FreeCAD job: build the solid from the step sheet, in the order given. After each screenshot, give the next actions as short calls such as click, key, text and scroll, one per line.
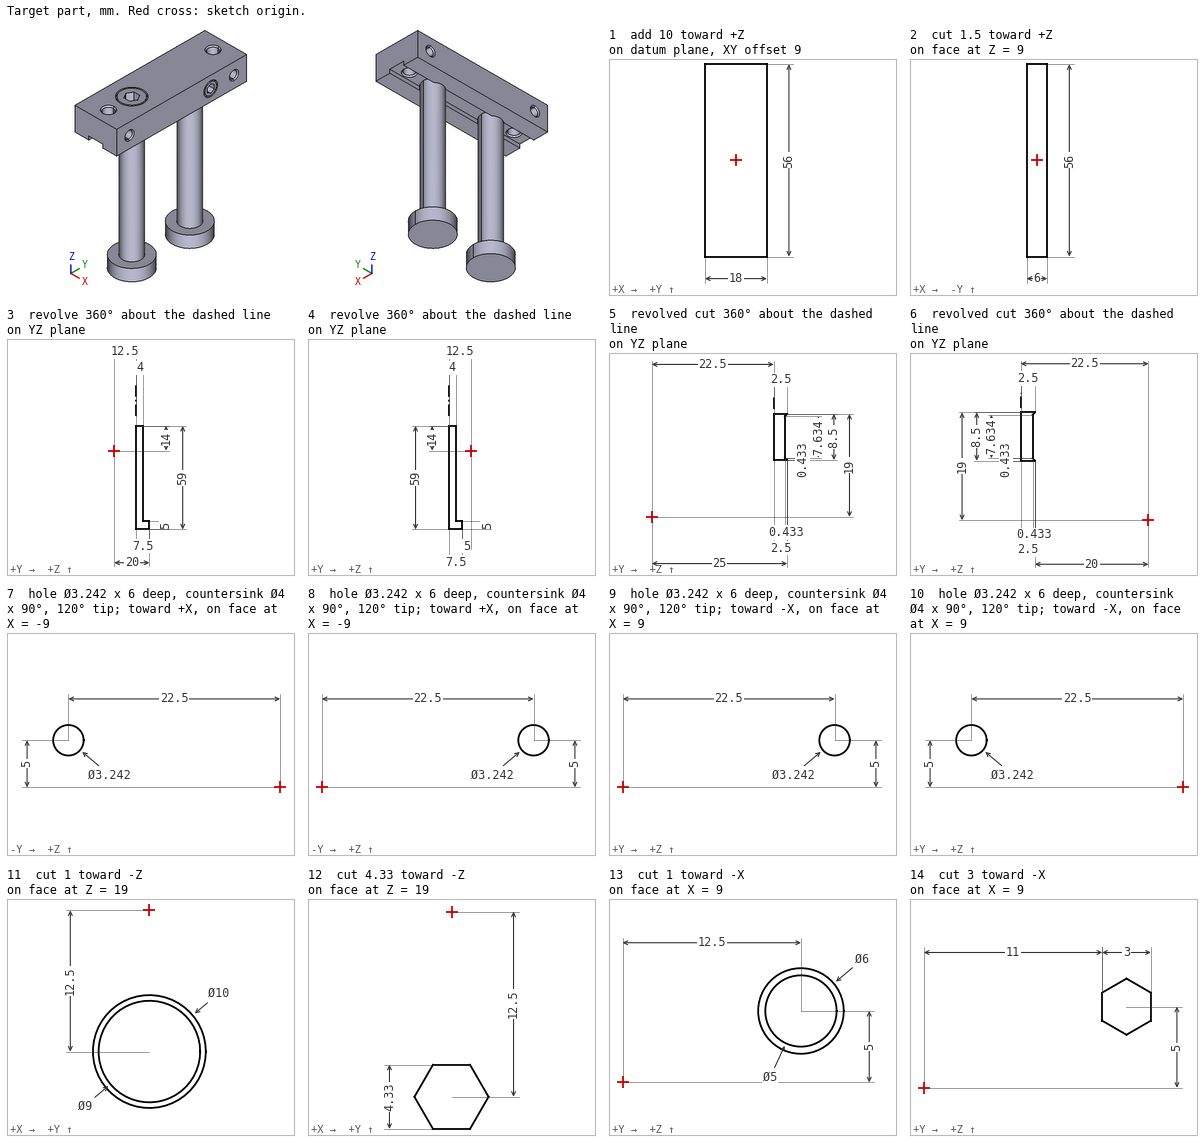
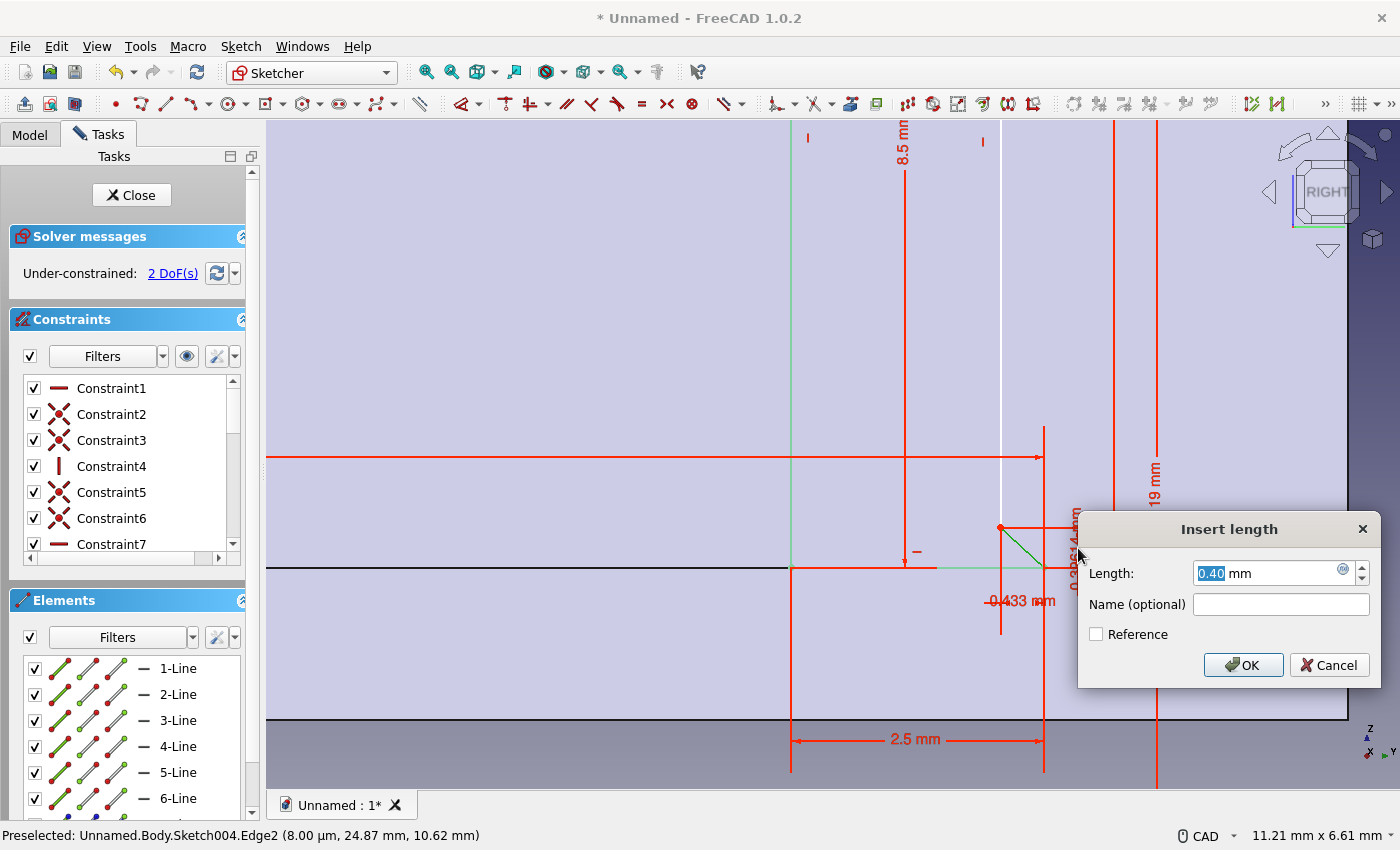
text(0.433)
key(Return)
key(Escape)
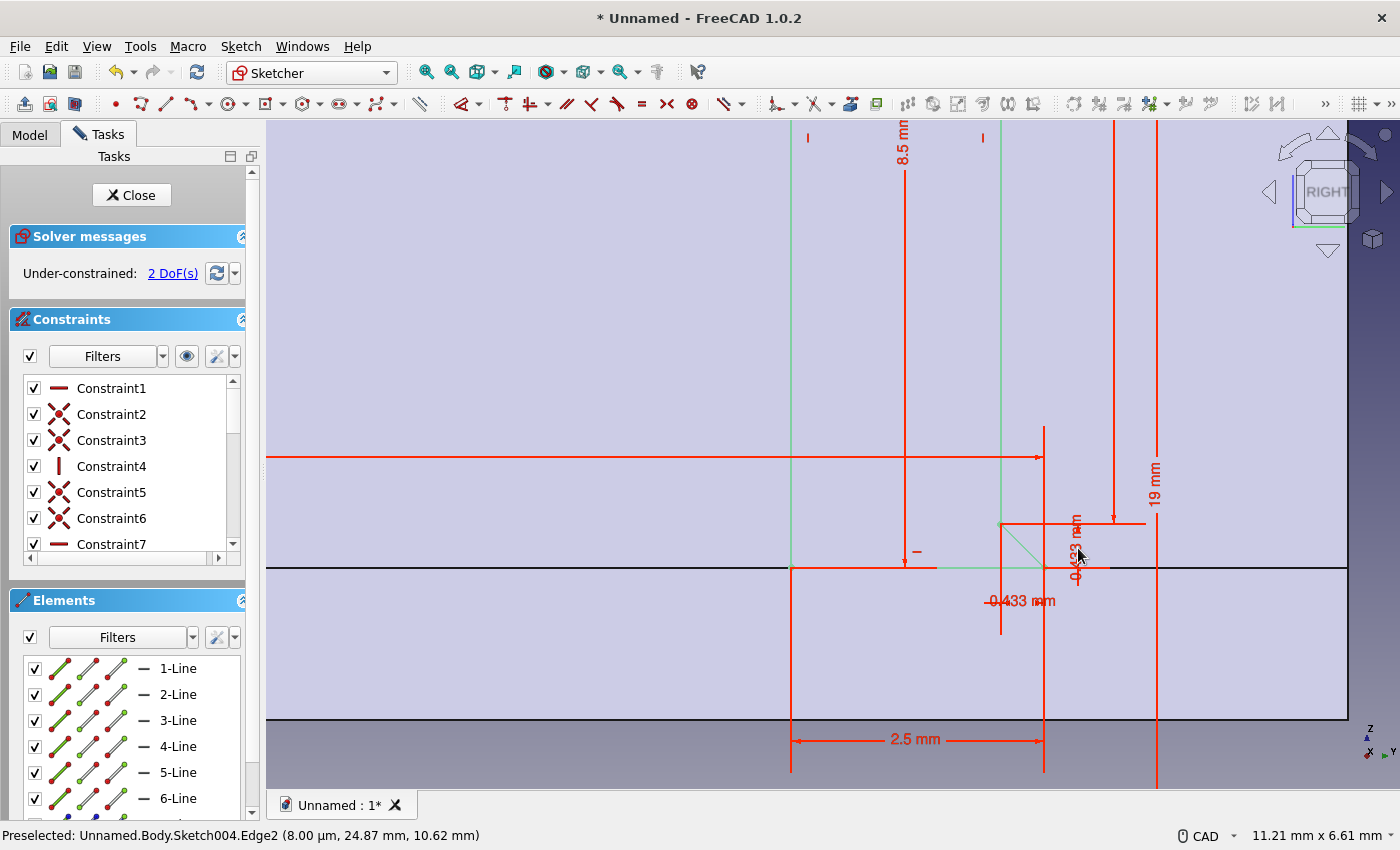
click(132, 195)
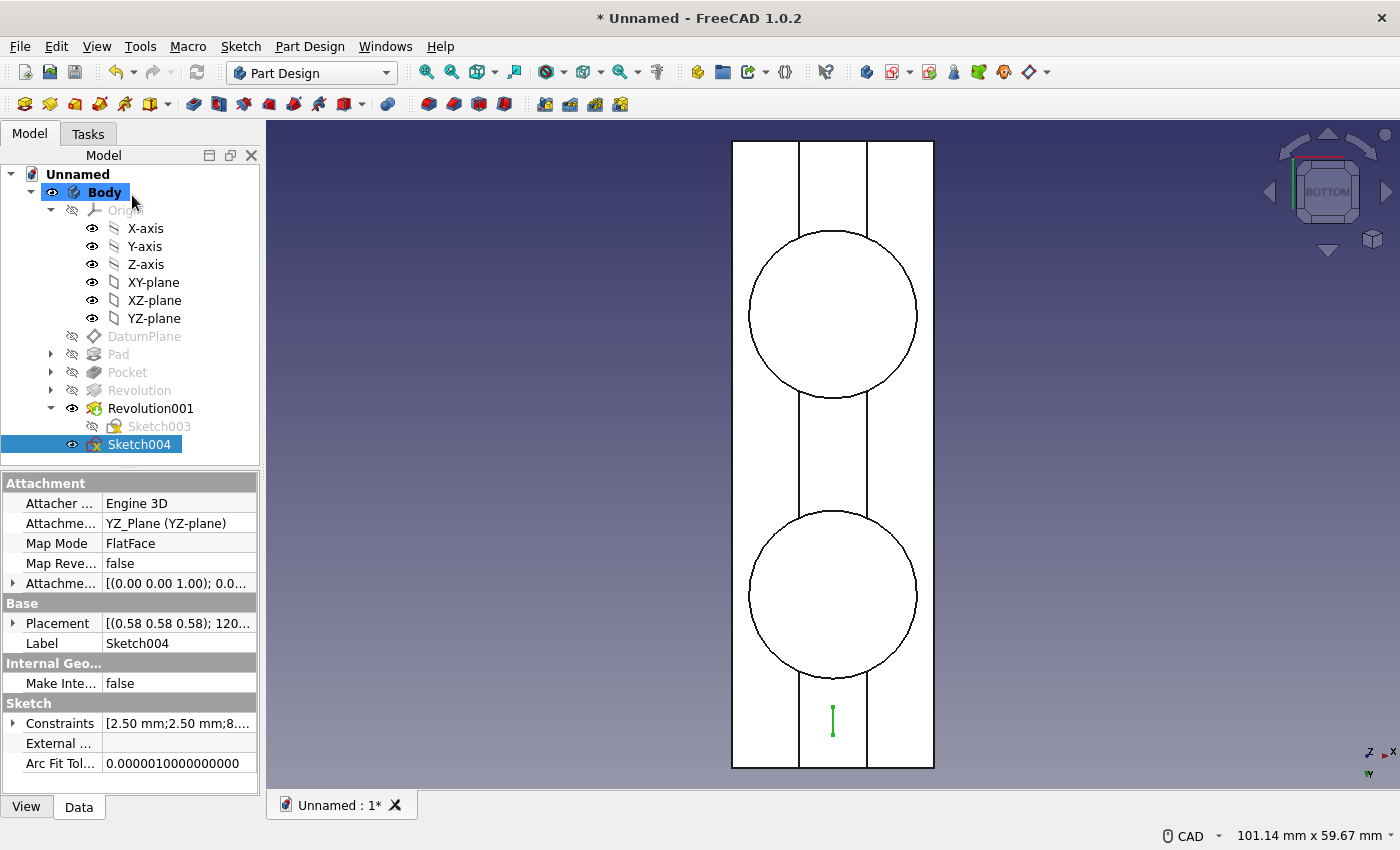
click(244, 104)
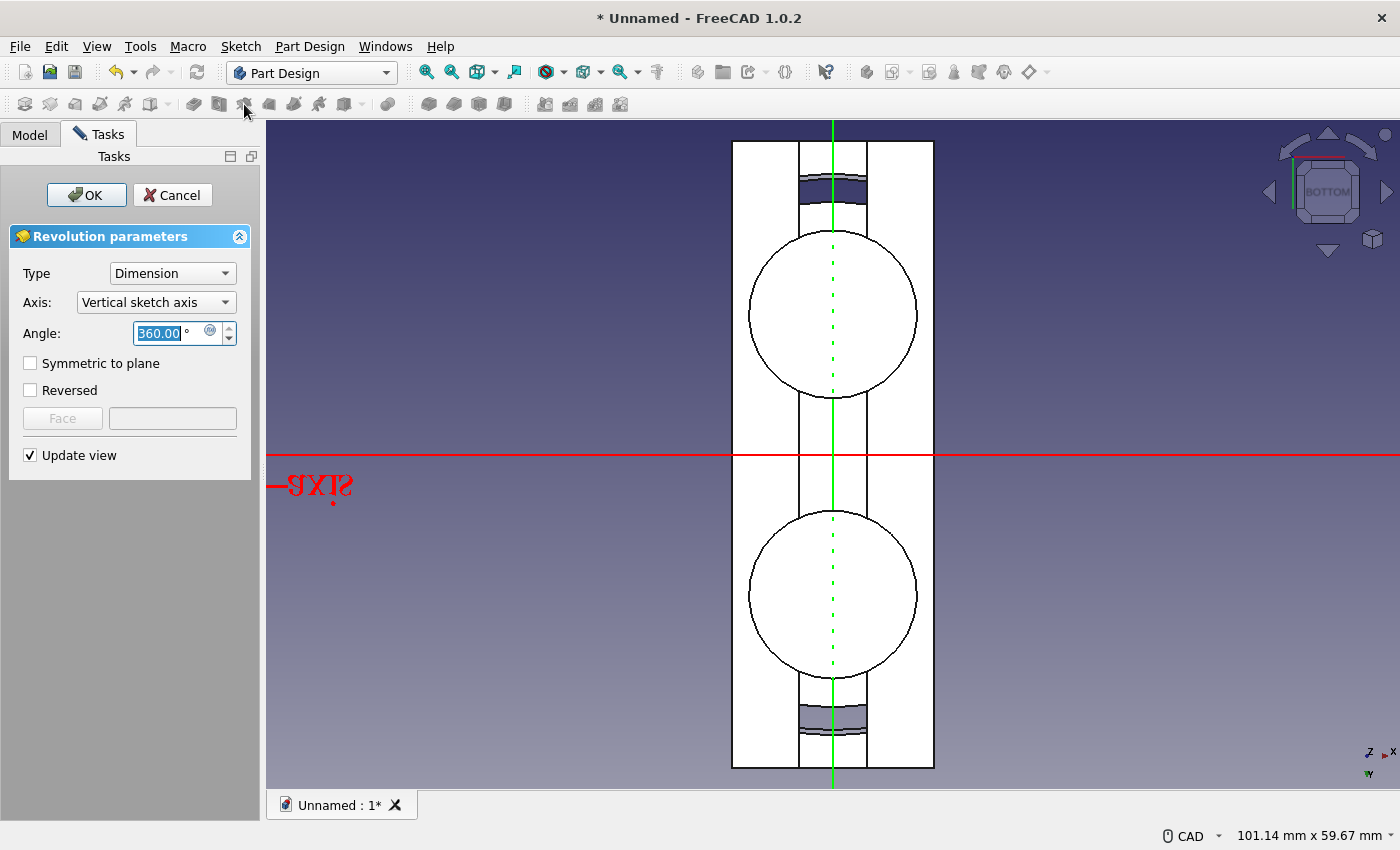
click(157, 302)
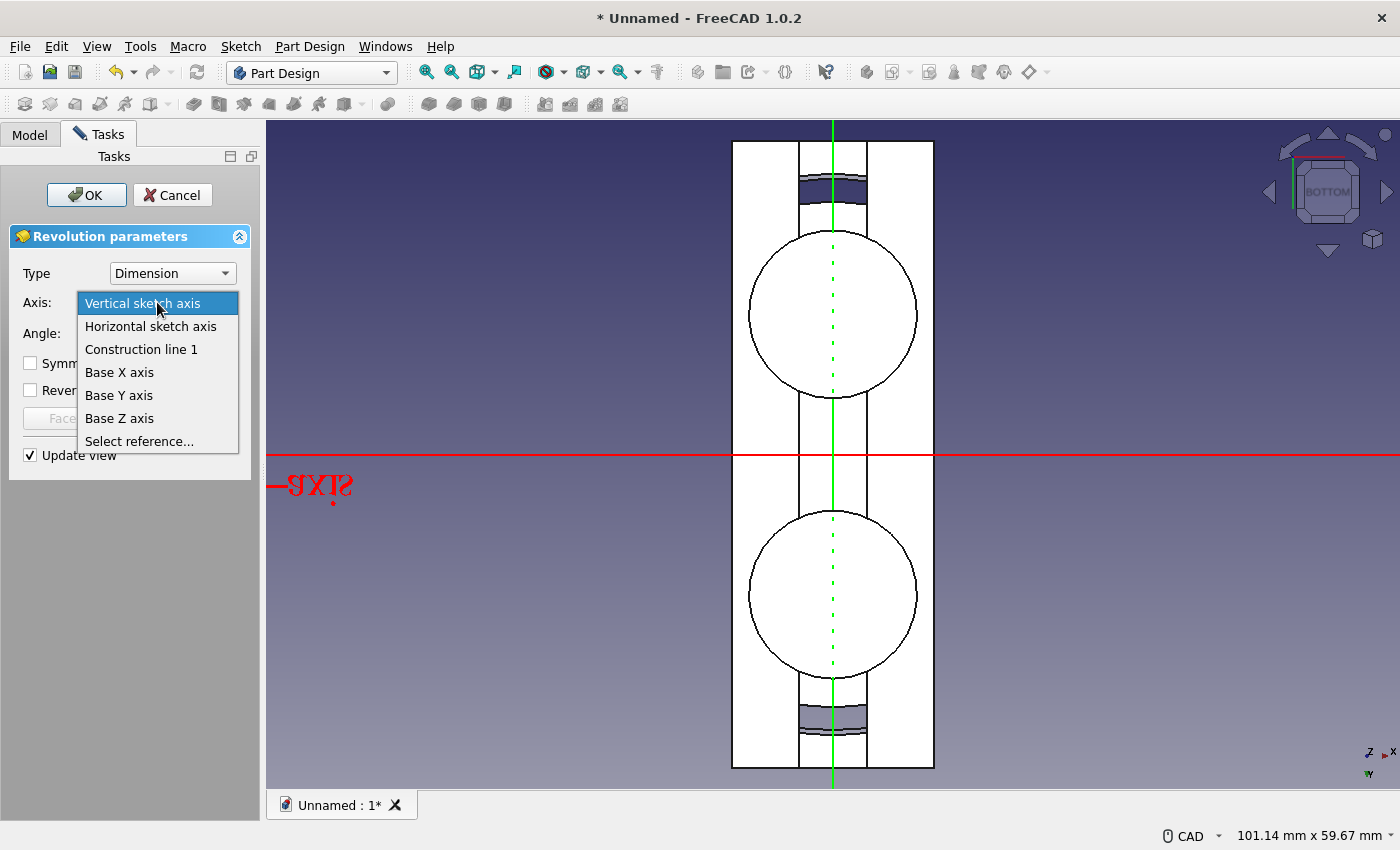
click(156, 350)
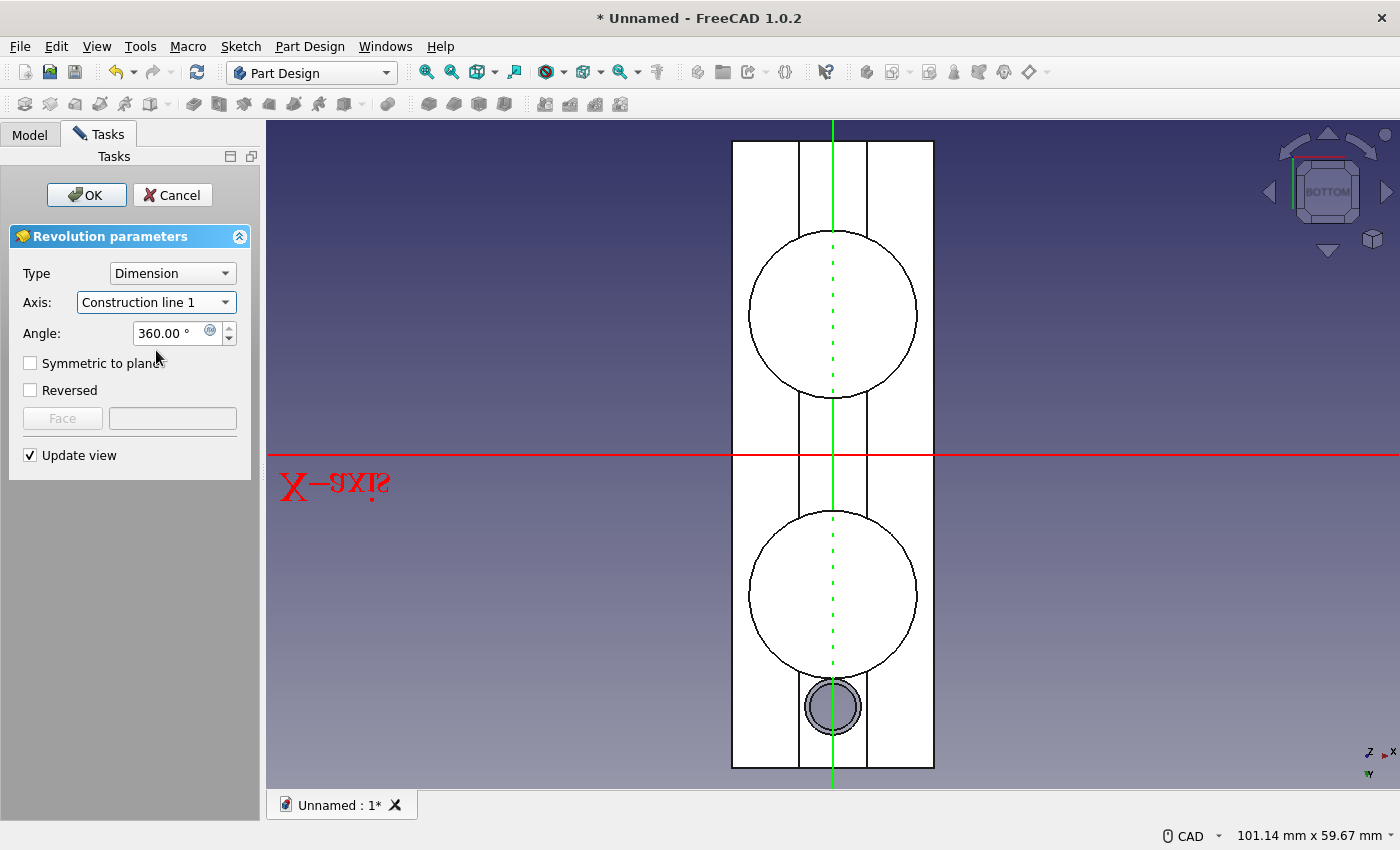
click(87, 195)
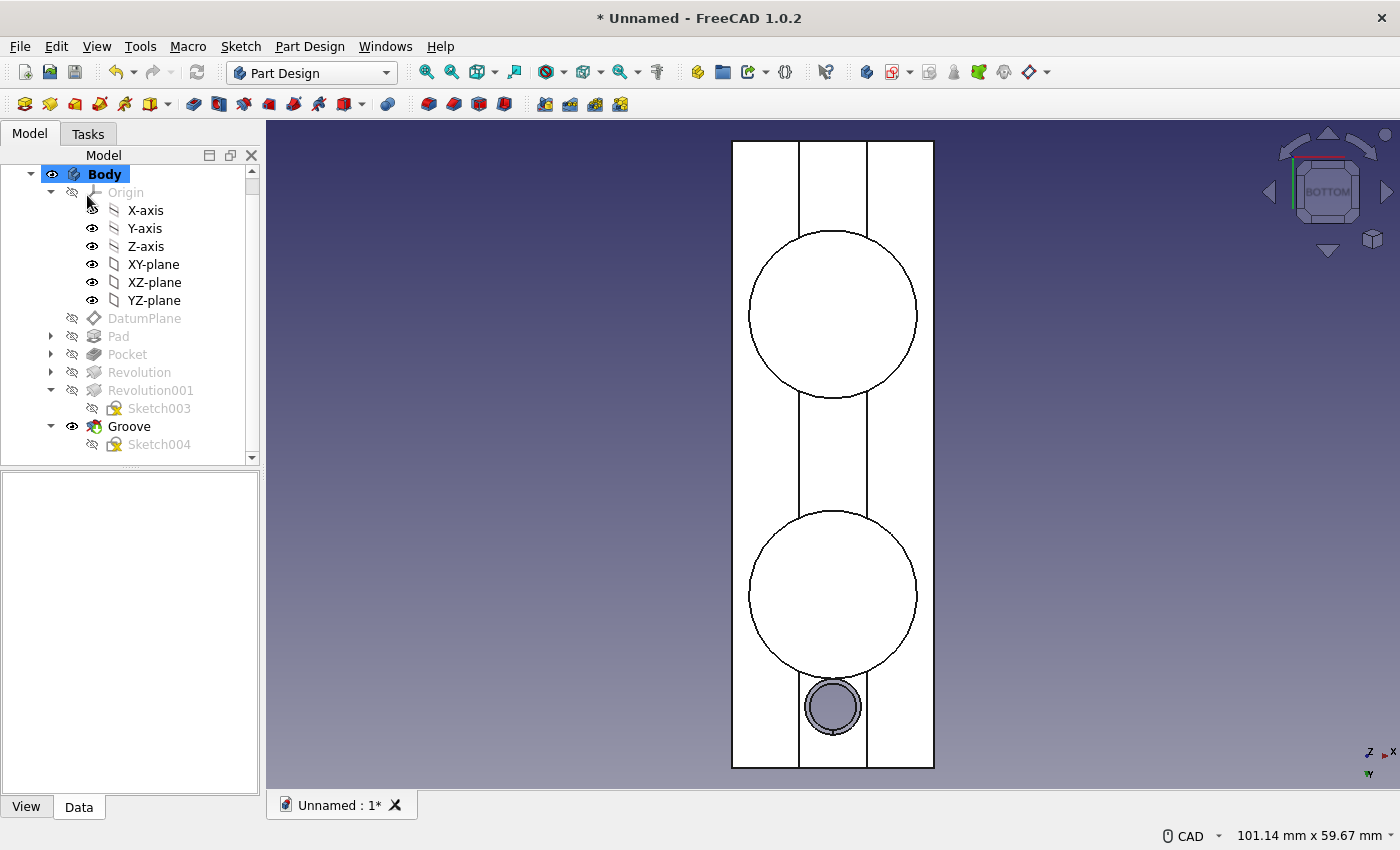
click(892, 72)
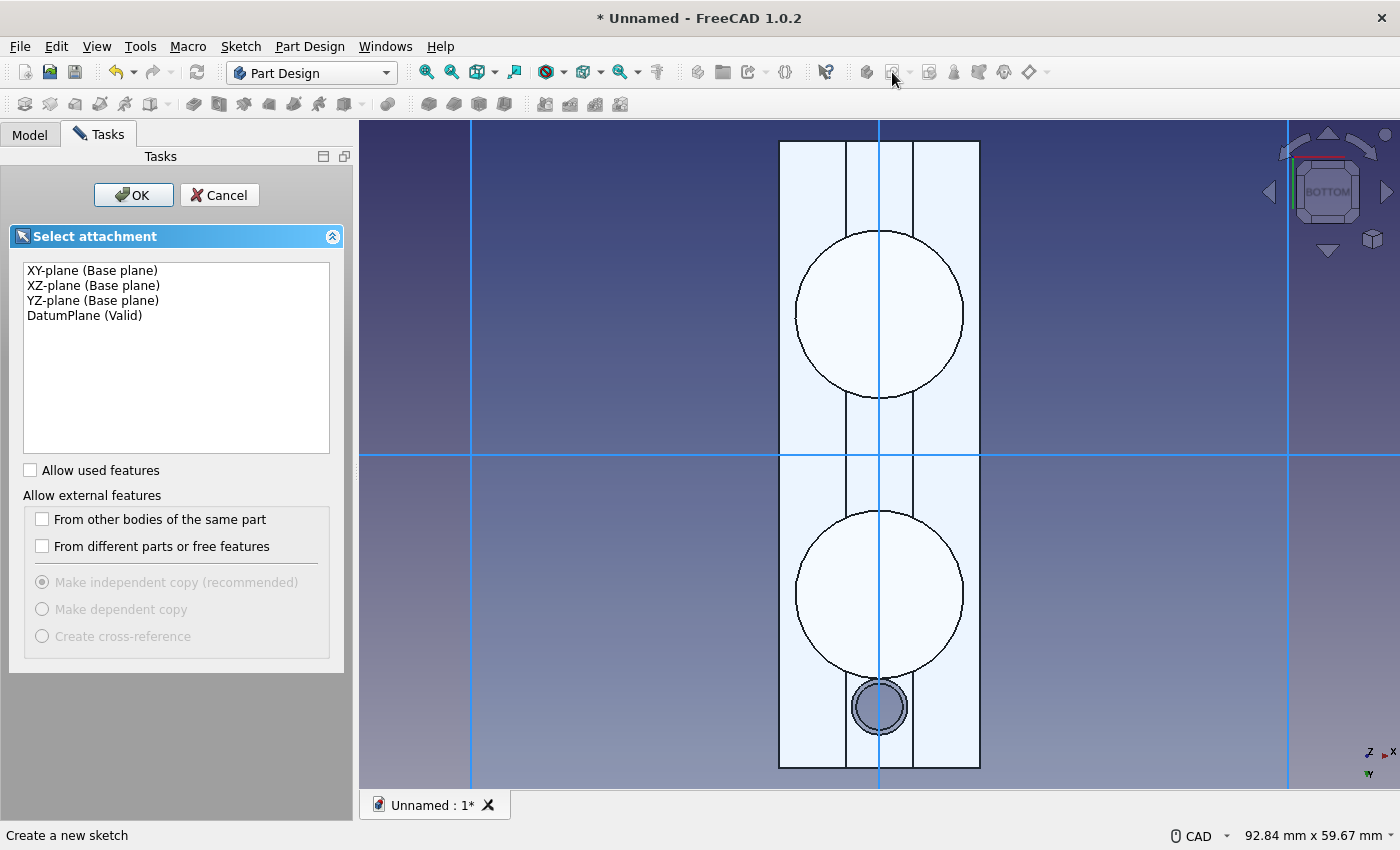
click(84, 300)